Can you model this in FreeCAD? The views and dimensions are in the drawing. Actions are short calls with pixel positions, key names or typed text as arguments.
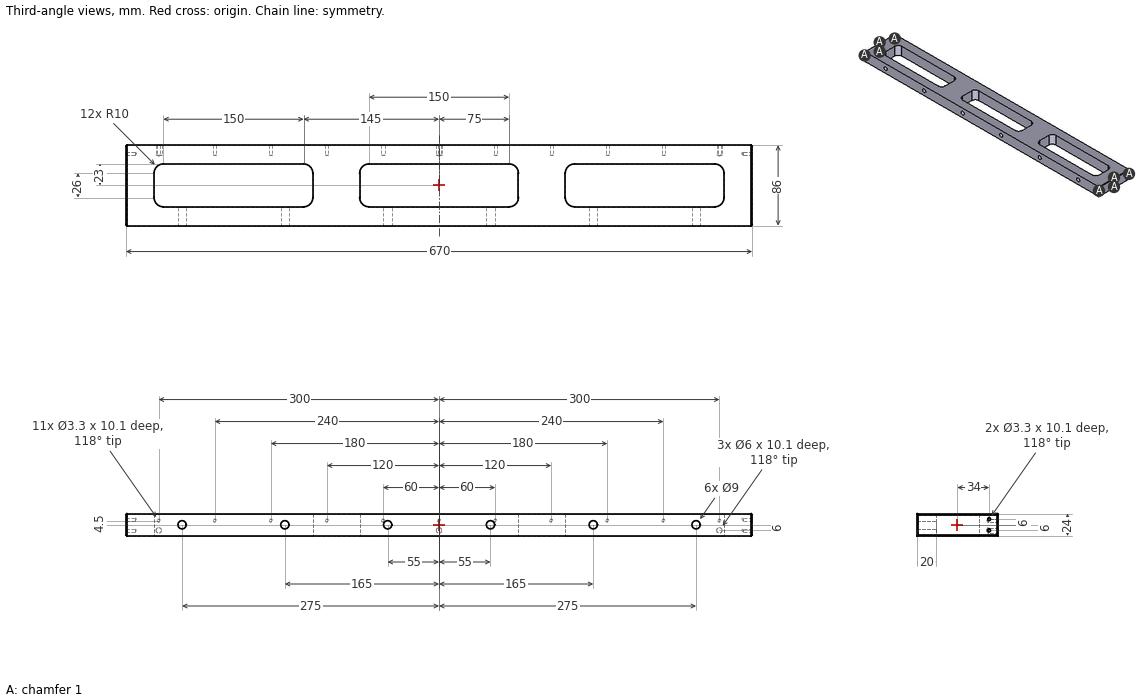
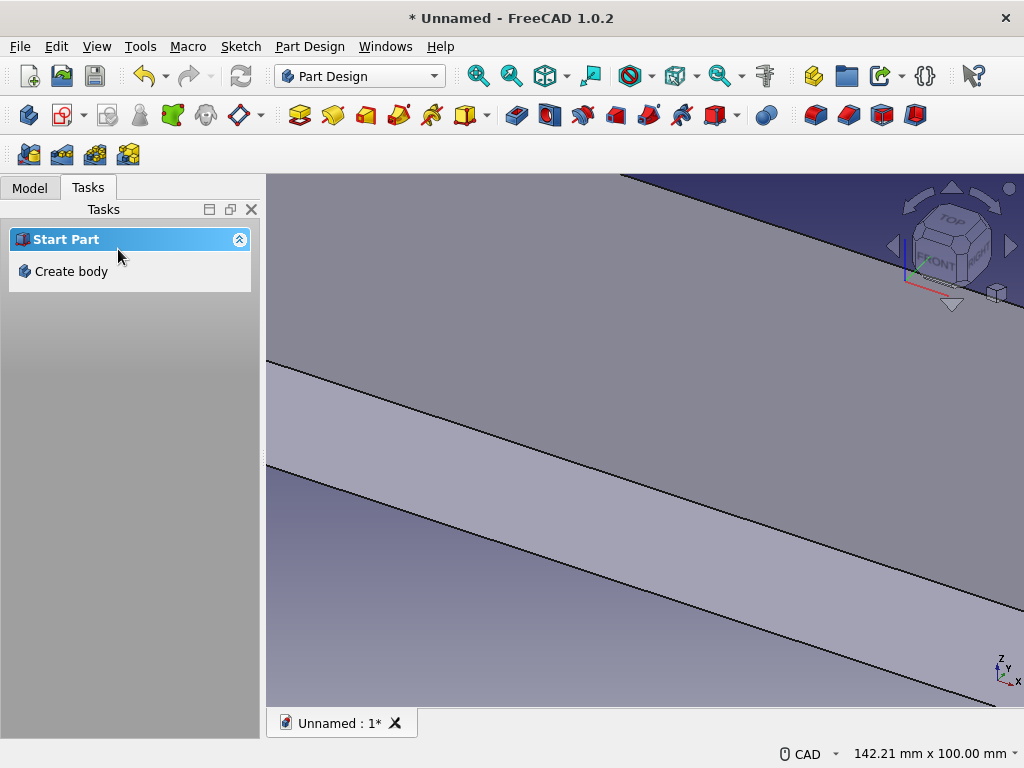
key(v)
key(f)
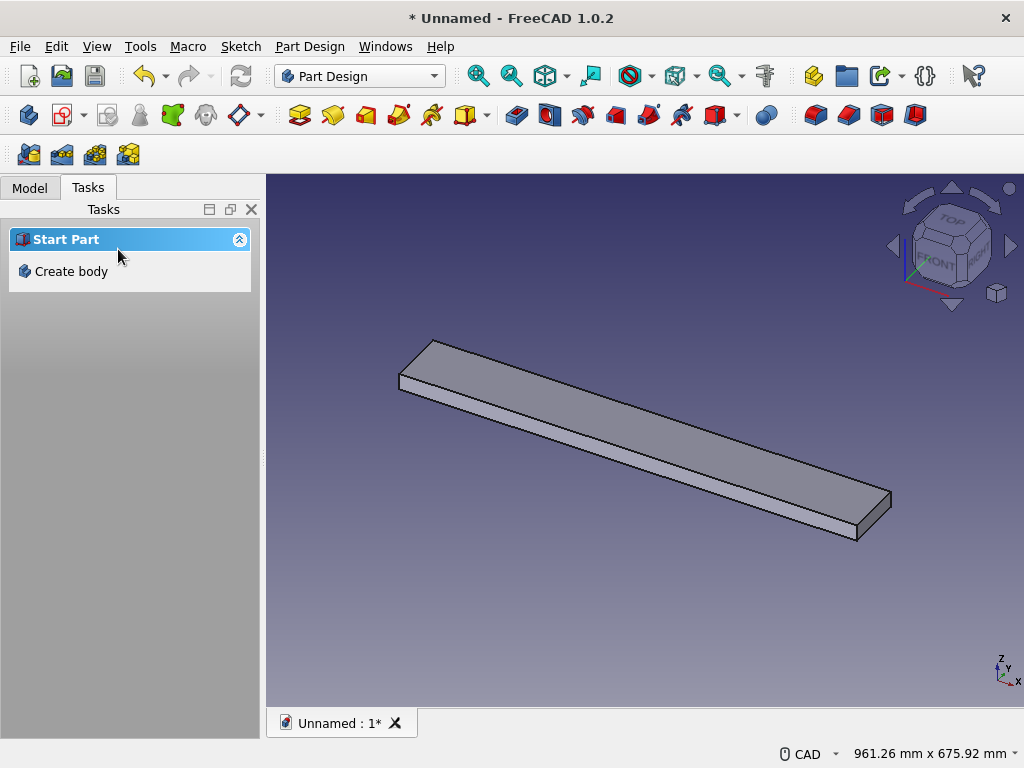
click(841, 497)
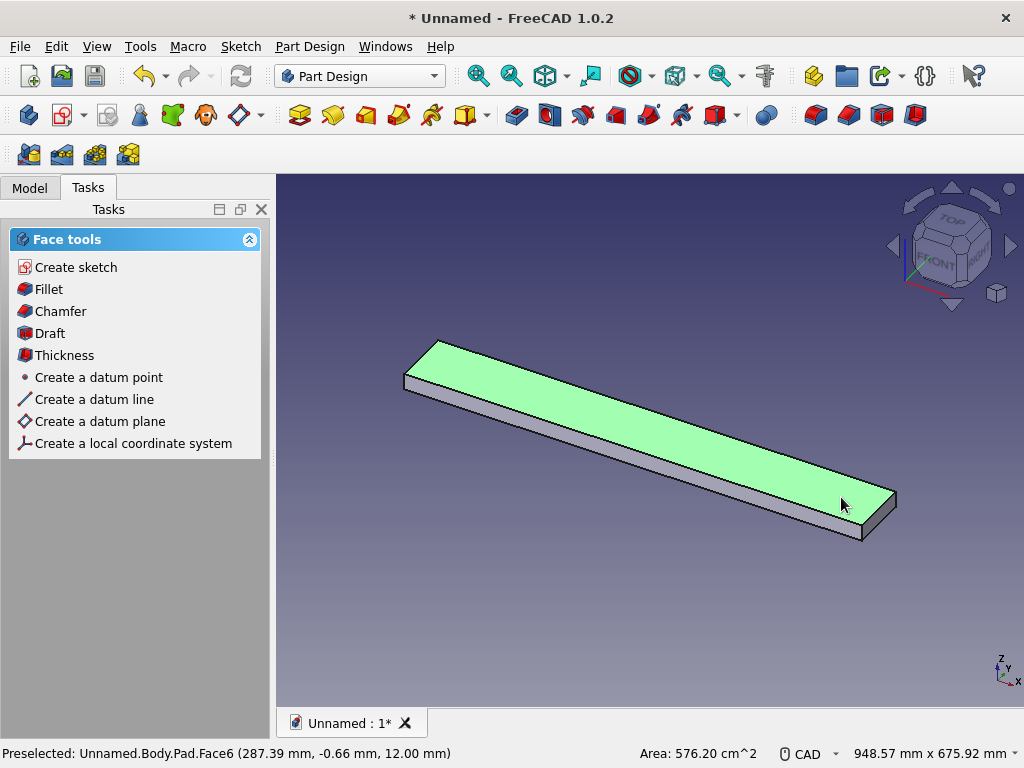
click(62, 116)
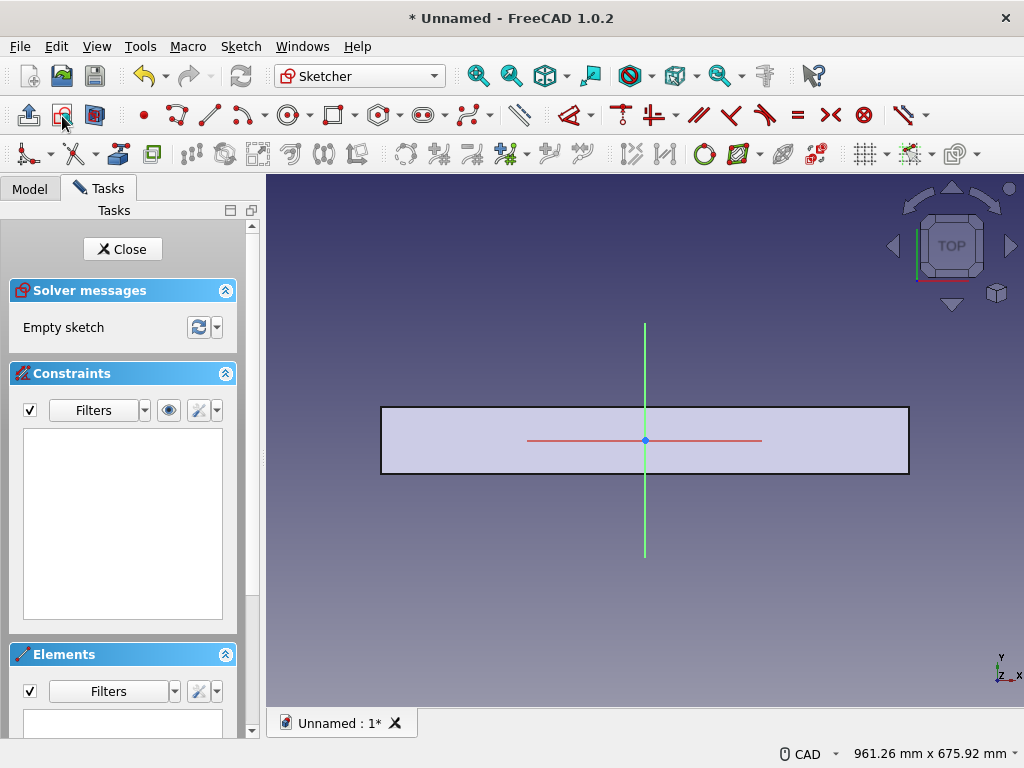
scroll(294, 440, down, 1)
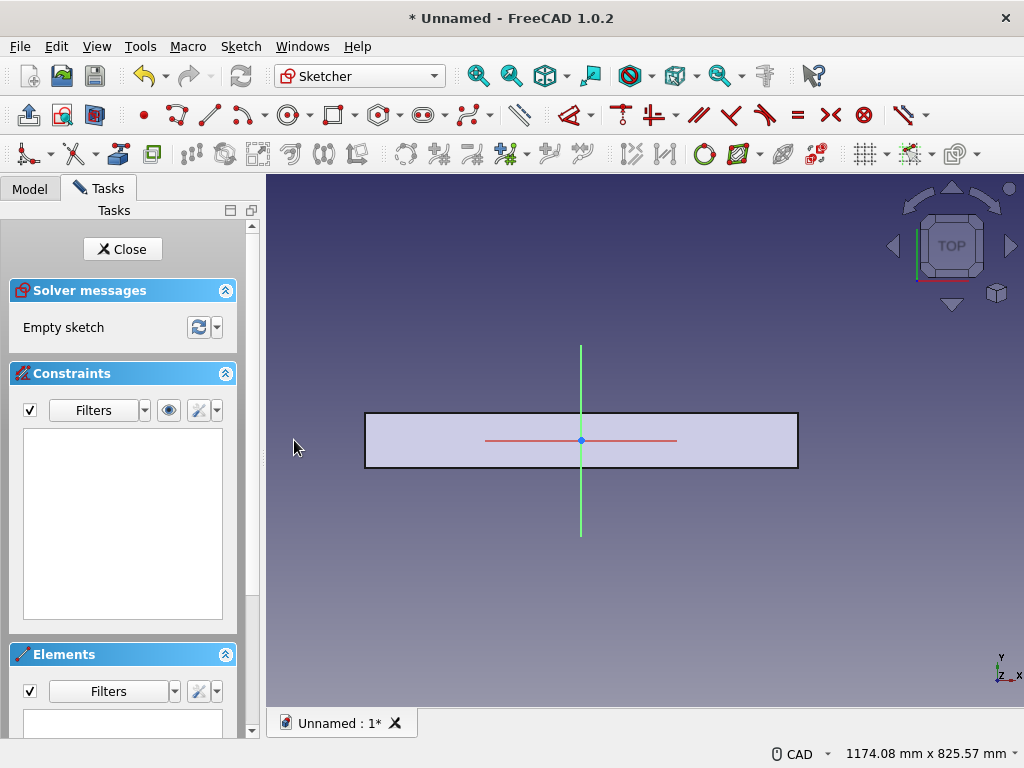
key(g)
key(l)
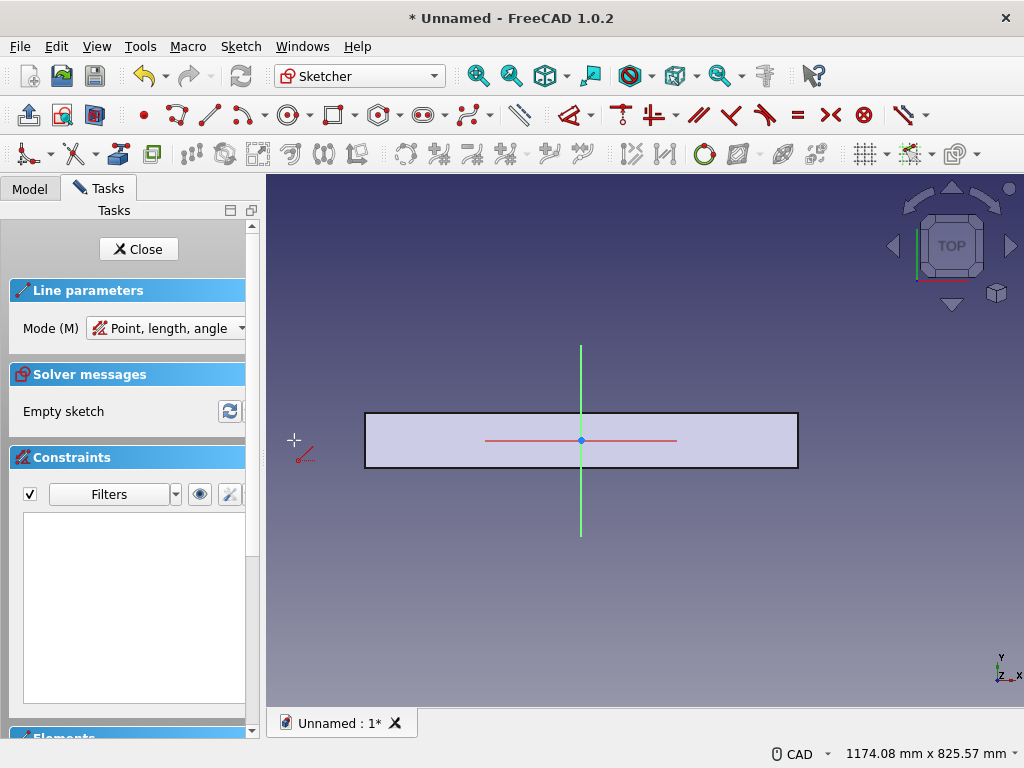
click(488, 426)
click(391, 426)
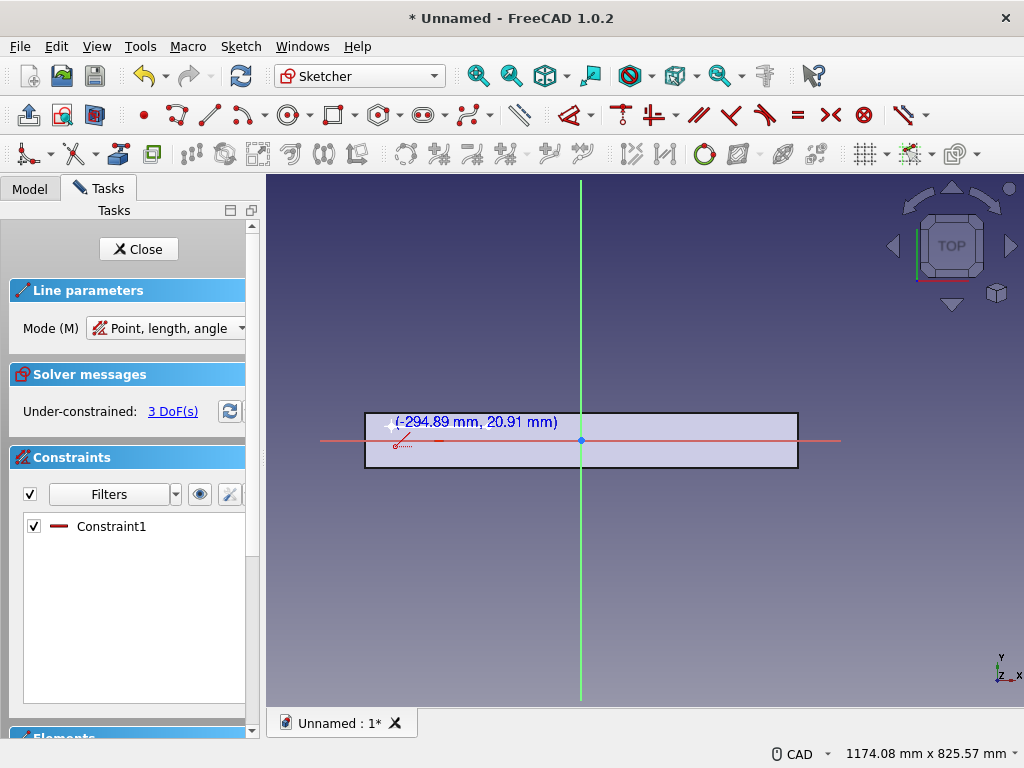
scroll(384, 432, up, 4)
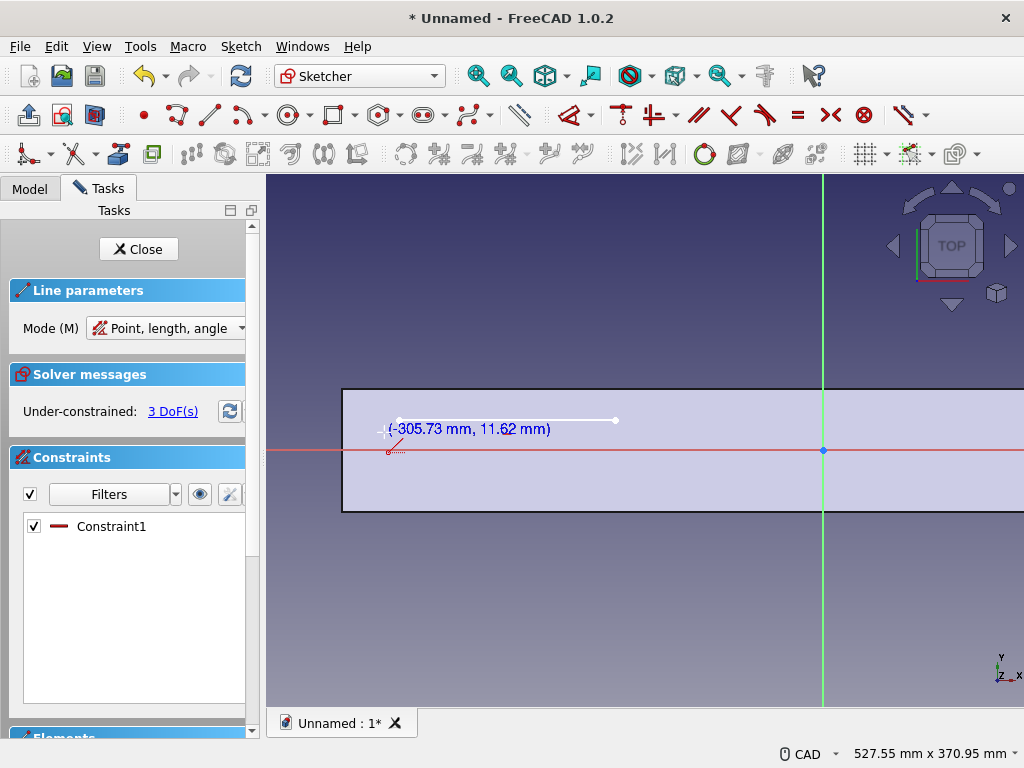
click(385, 432)
click(385, 469)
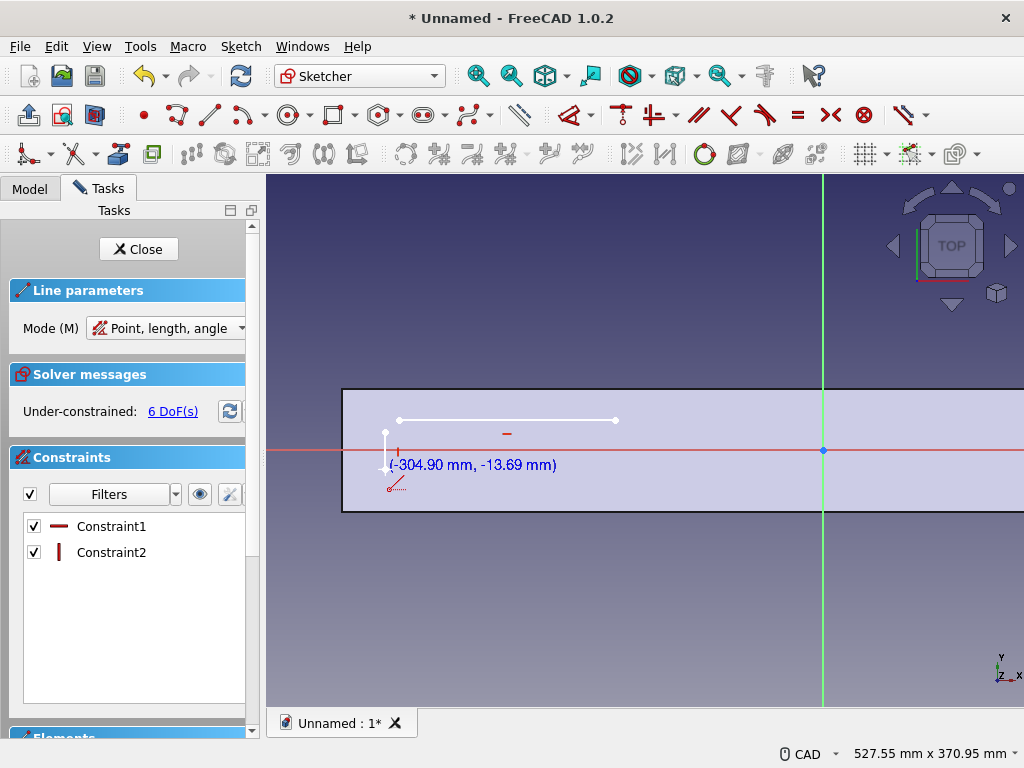
click(399, 483)
click(615, 483)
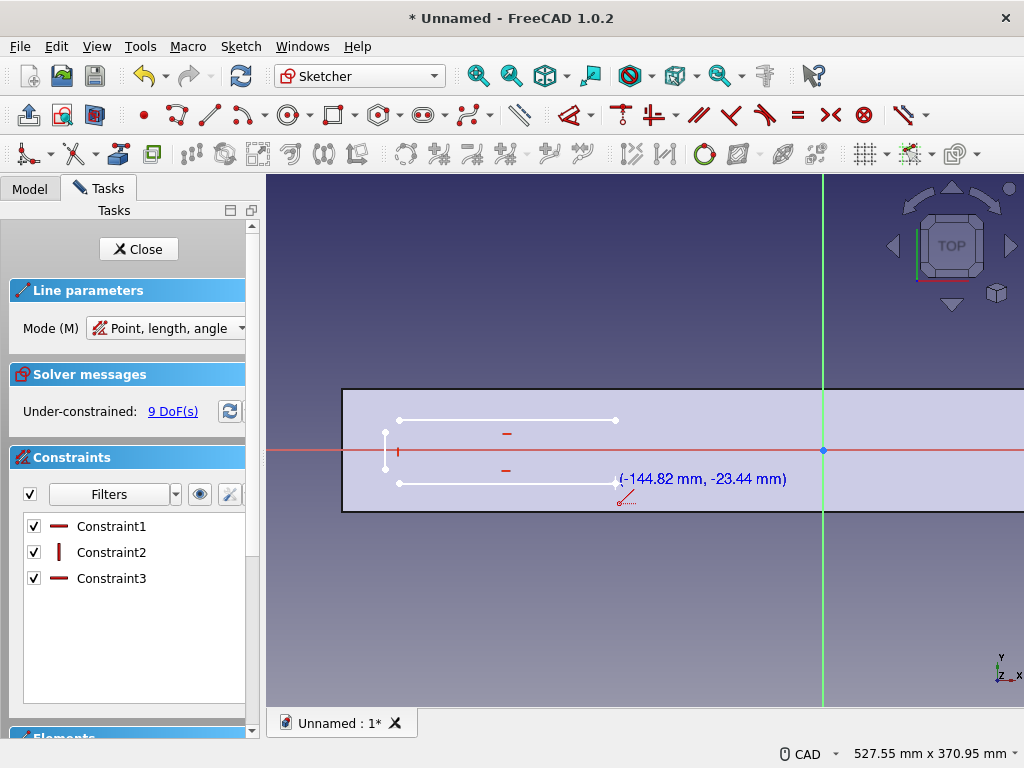
click(629, 469)
click(629, 432)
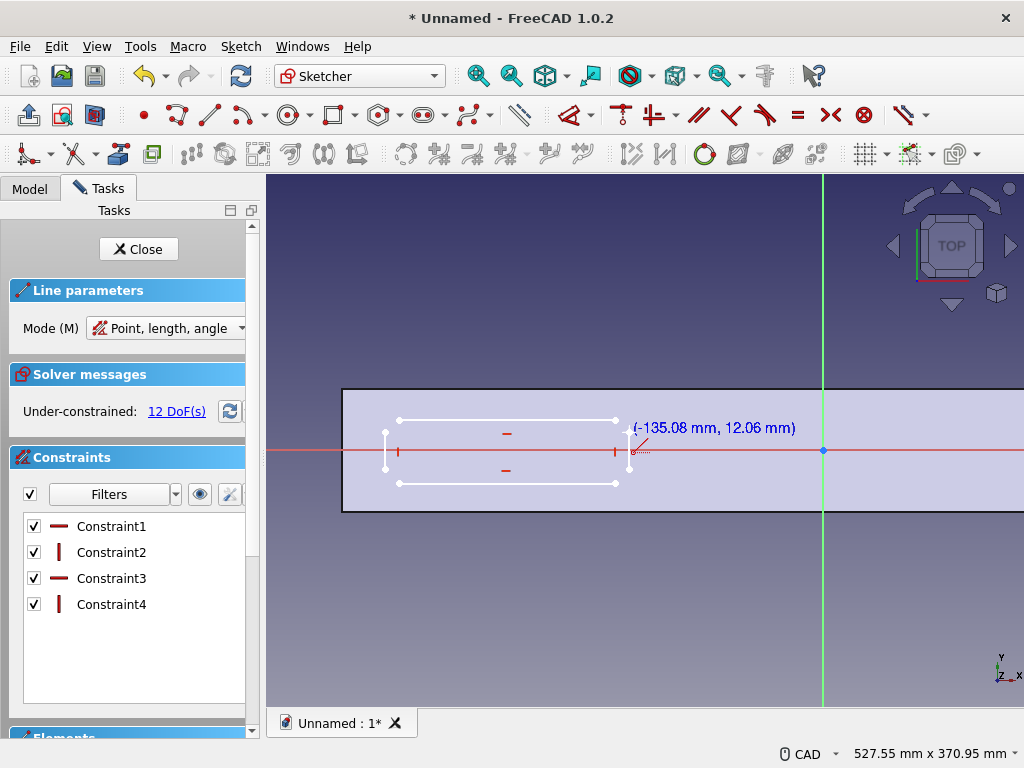
click(264, 116)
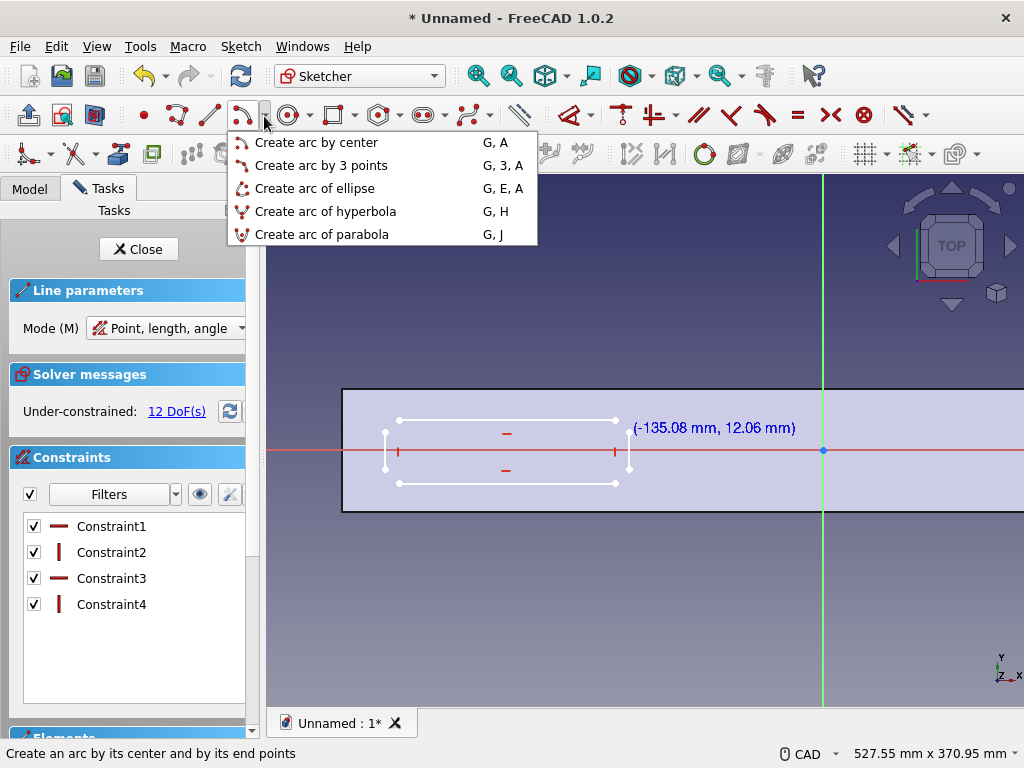
click(382, 166)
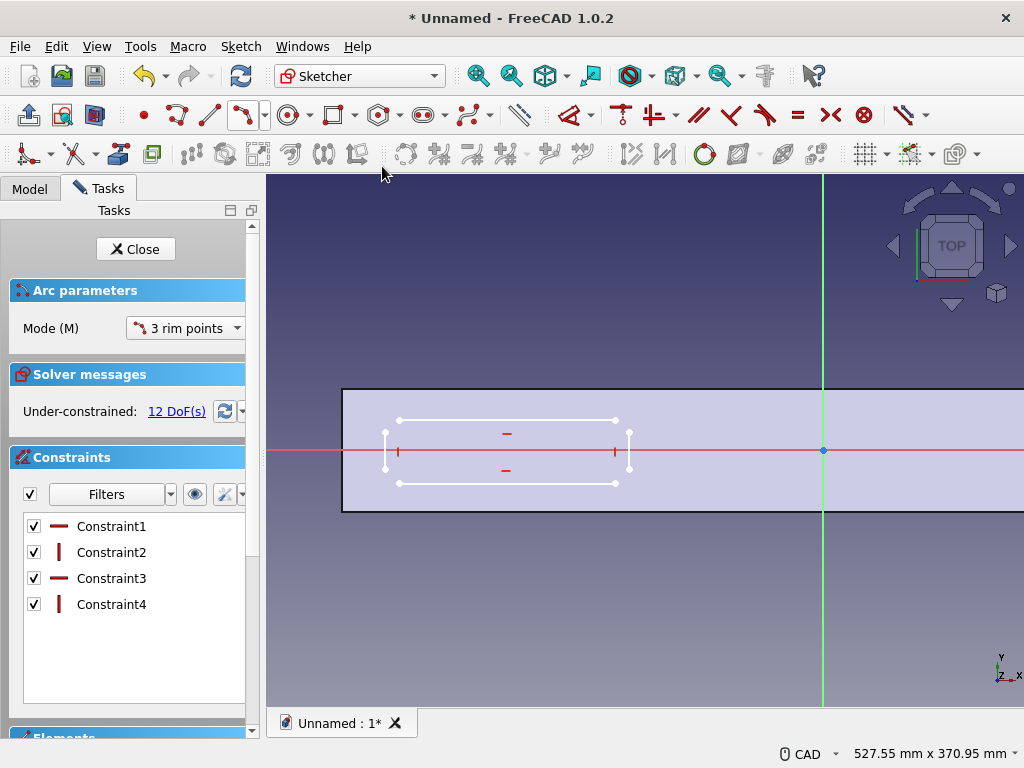
click(399, 420)
click(385, 433)